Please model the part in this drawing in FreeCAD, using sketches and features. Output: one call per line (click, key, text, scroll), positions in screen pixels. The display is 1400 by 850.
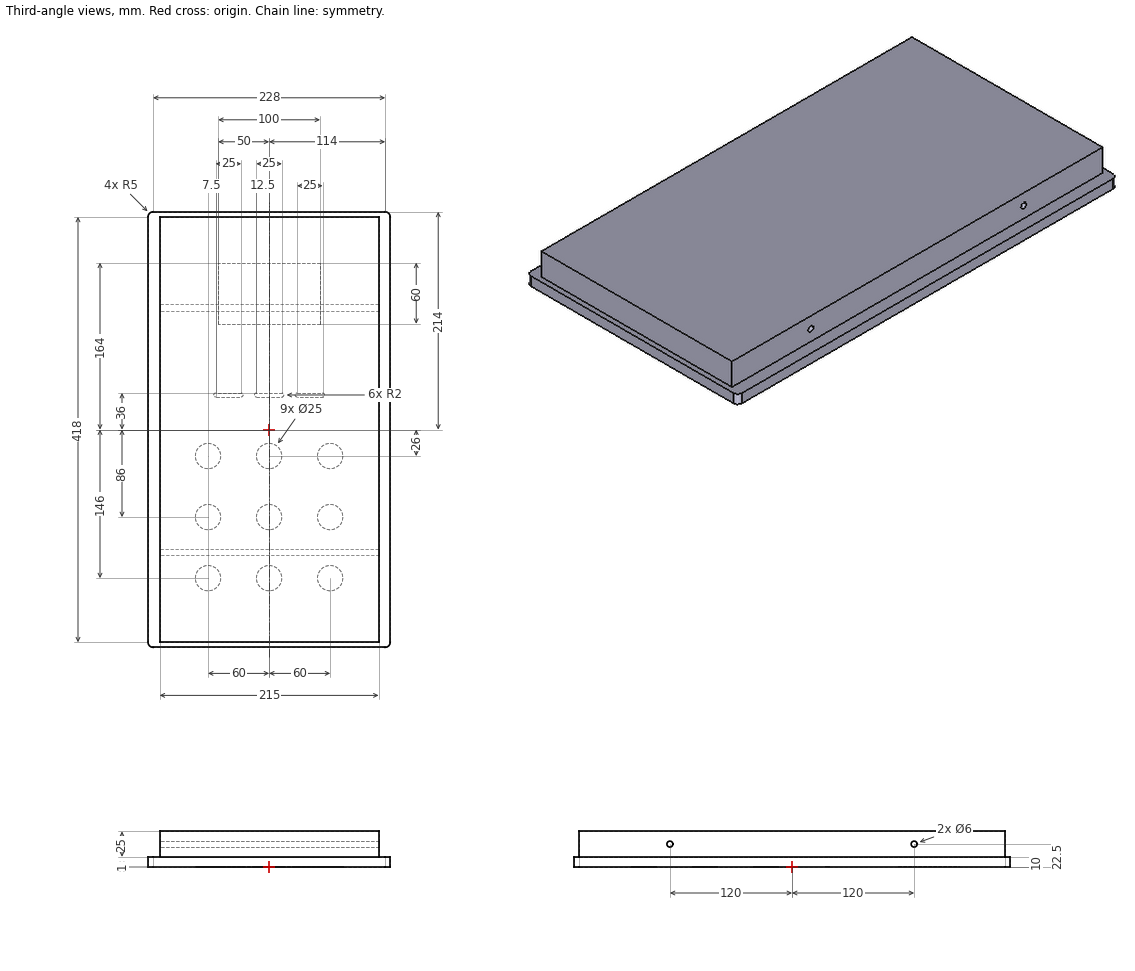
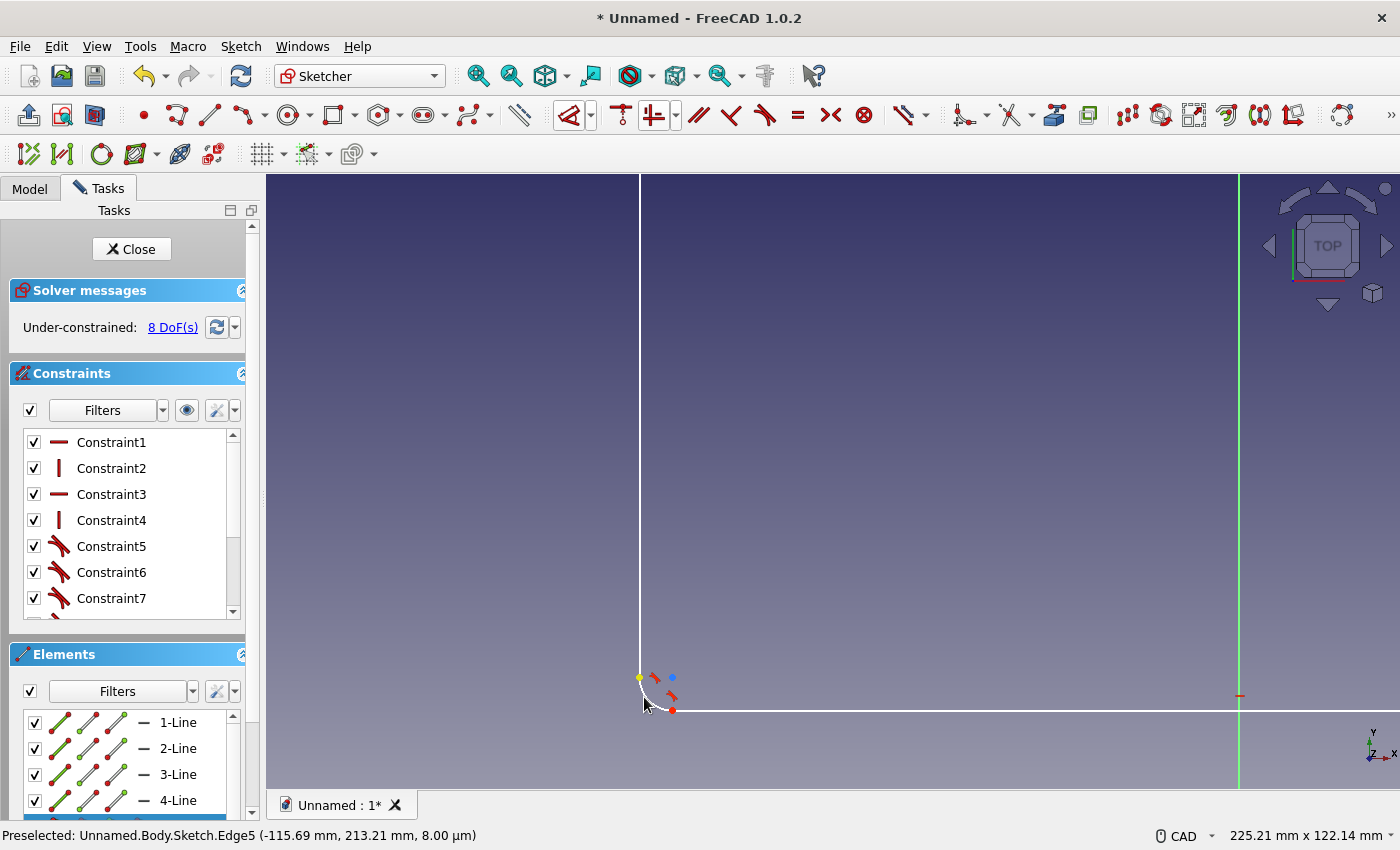
click(643, 692)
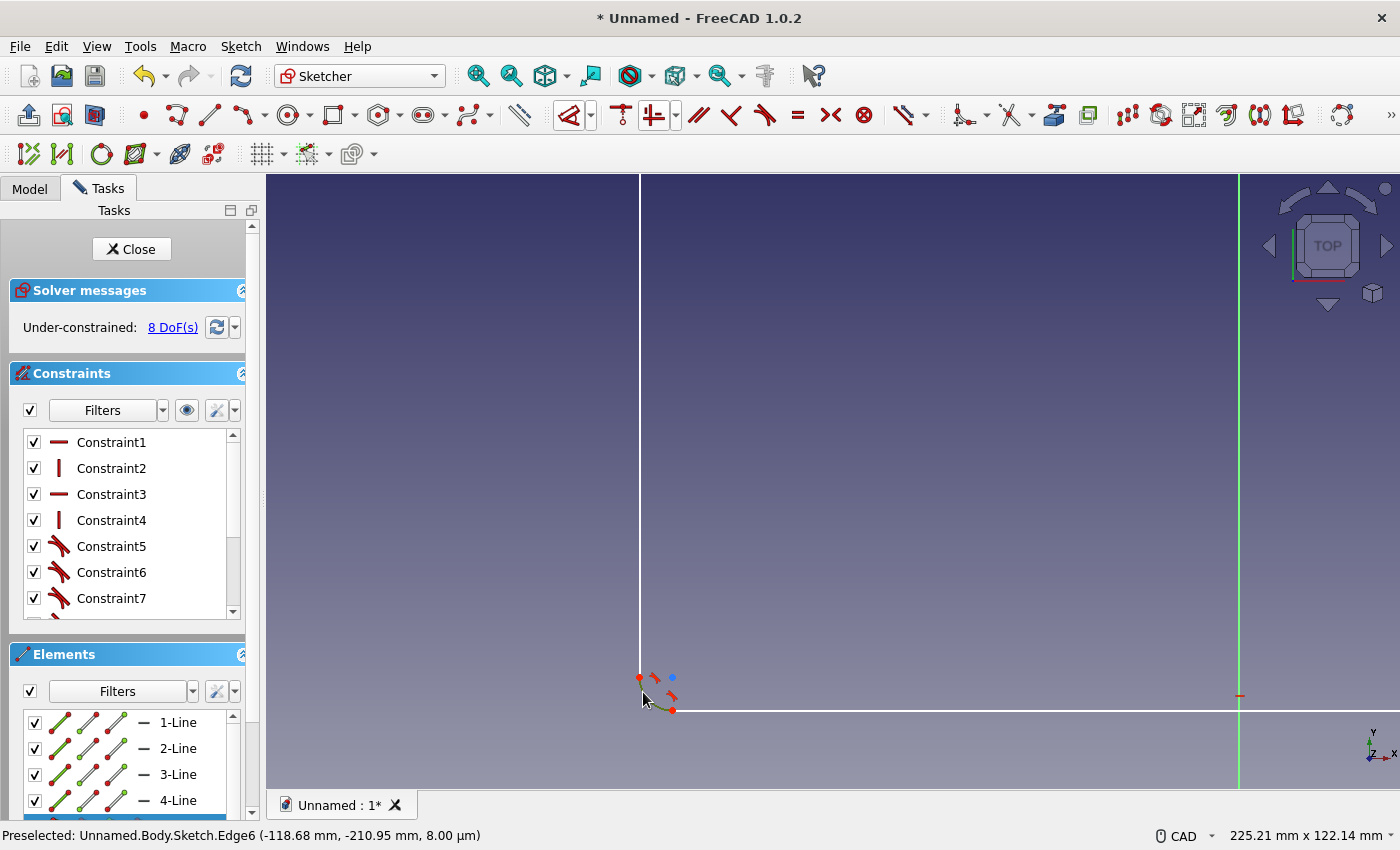
scroll(644, 698, down, 8)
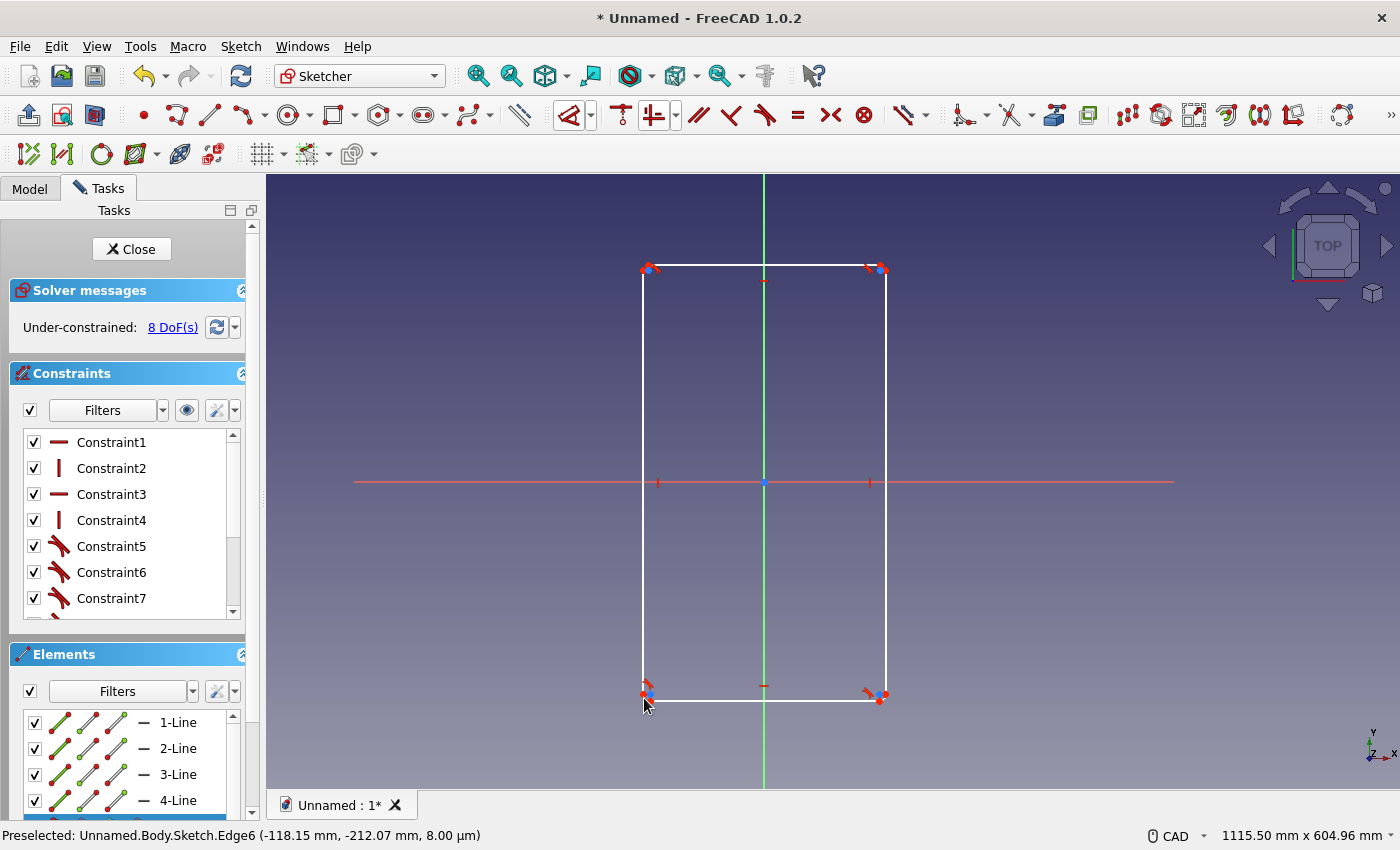
scroll(882, 701, up, 8)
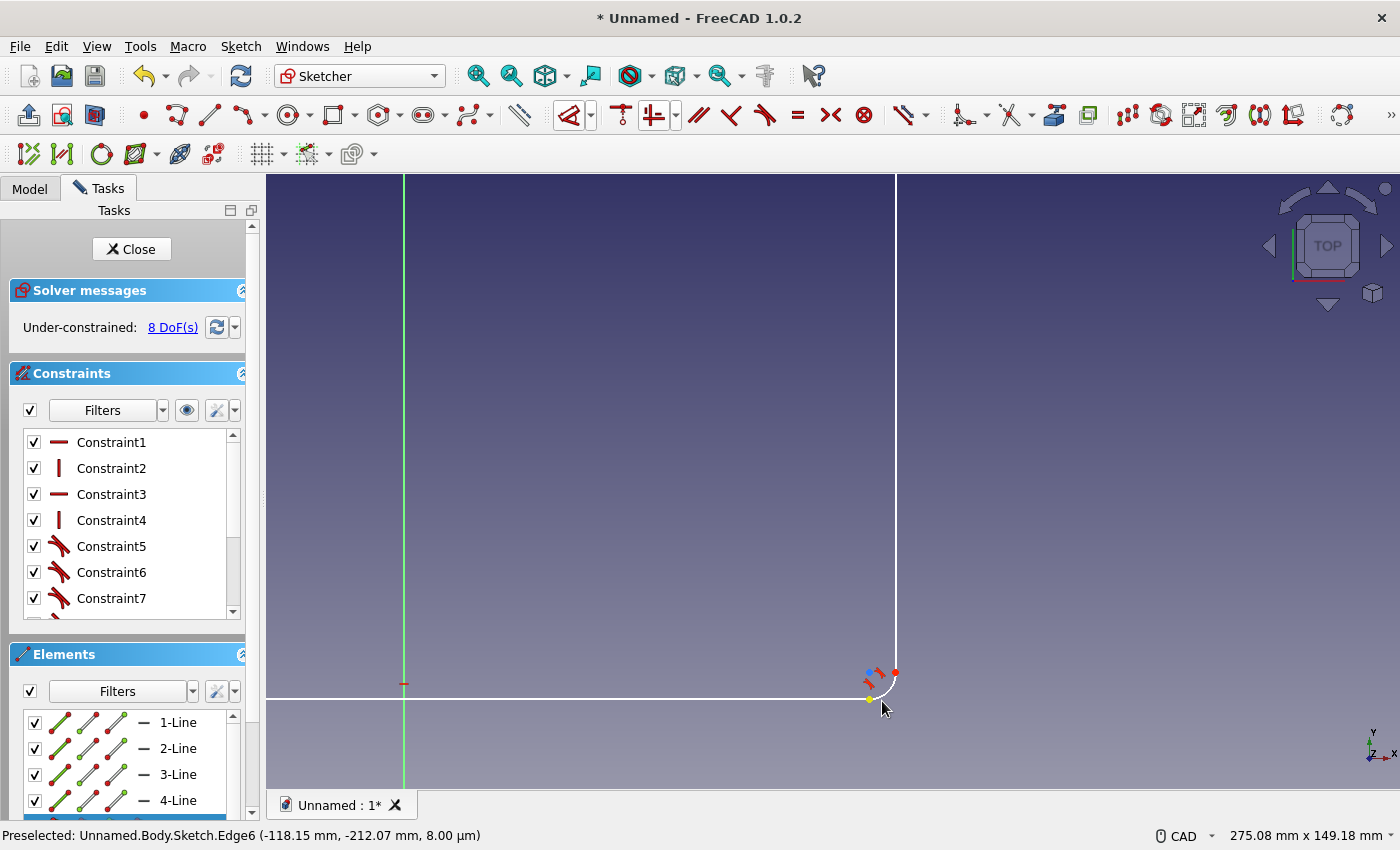
click(881, 695)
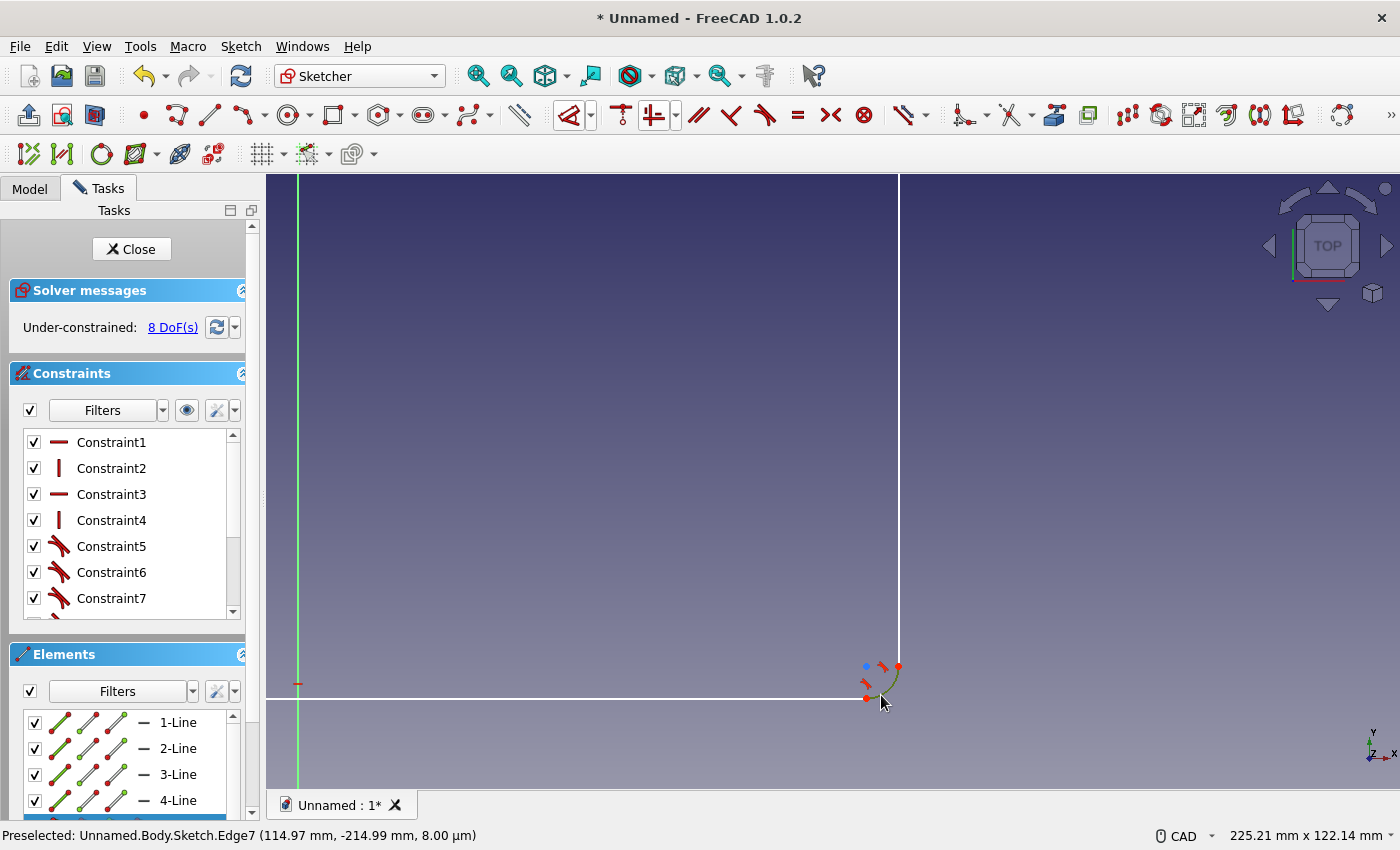
scroll(883, 701, down, 8)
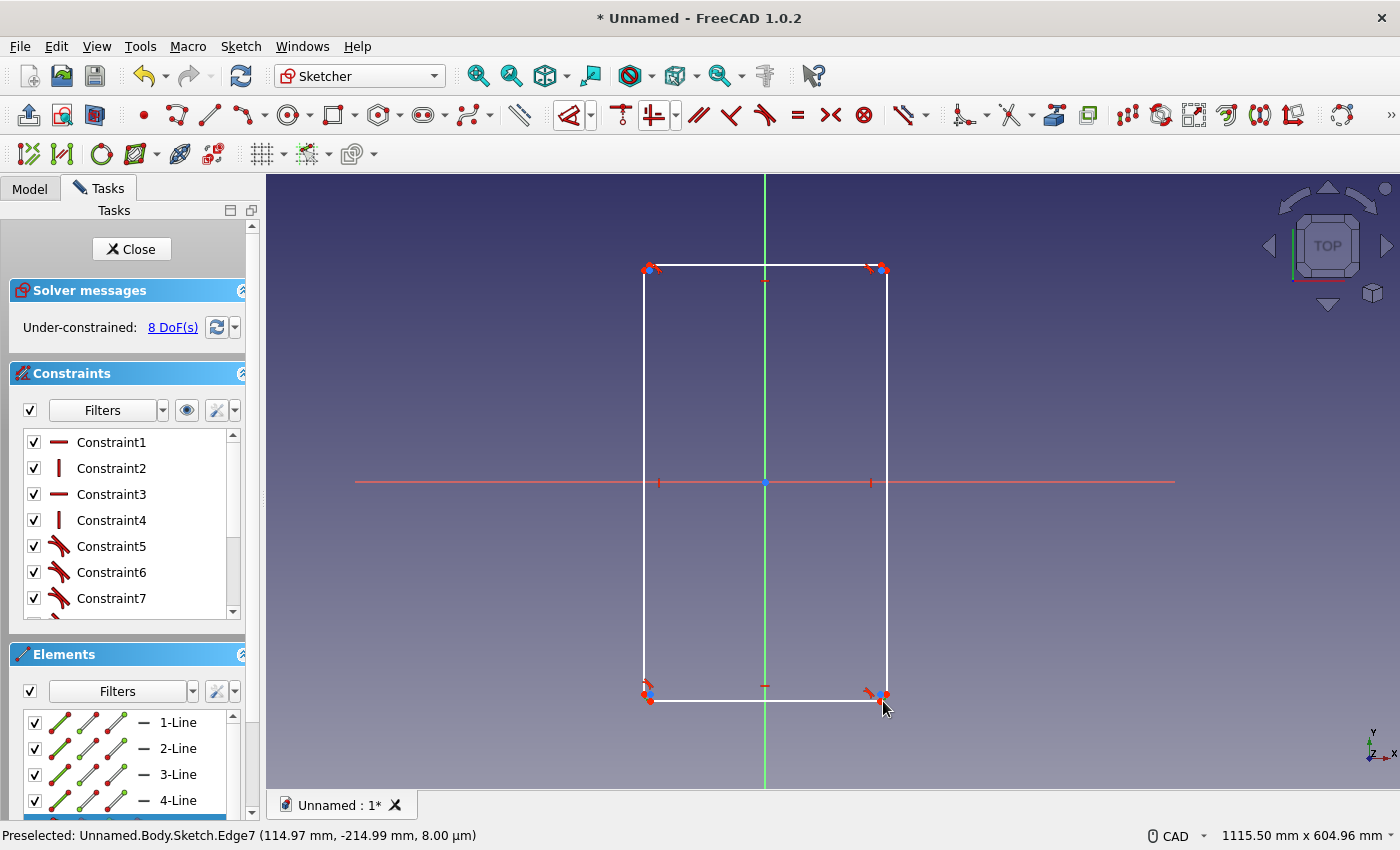
scroll(886, 268, up, 9)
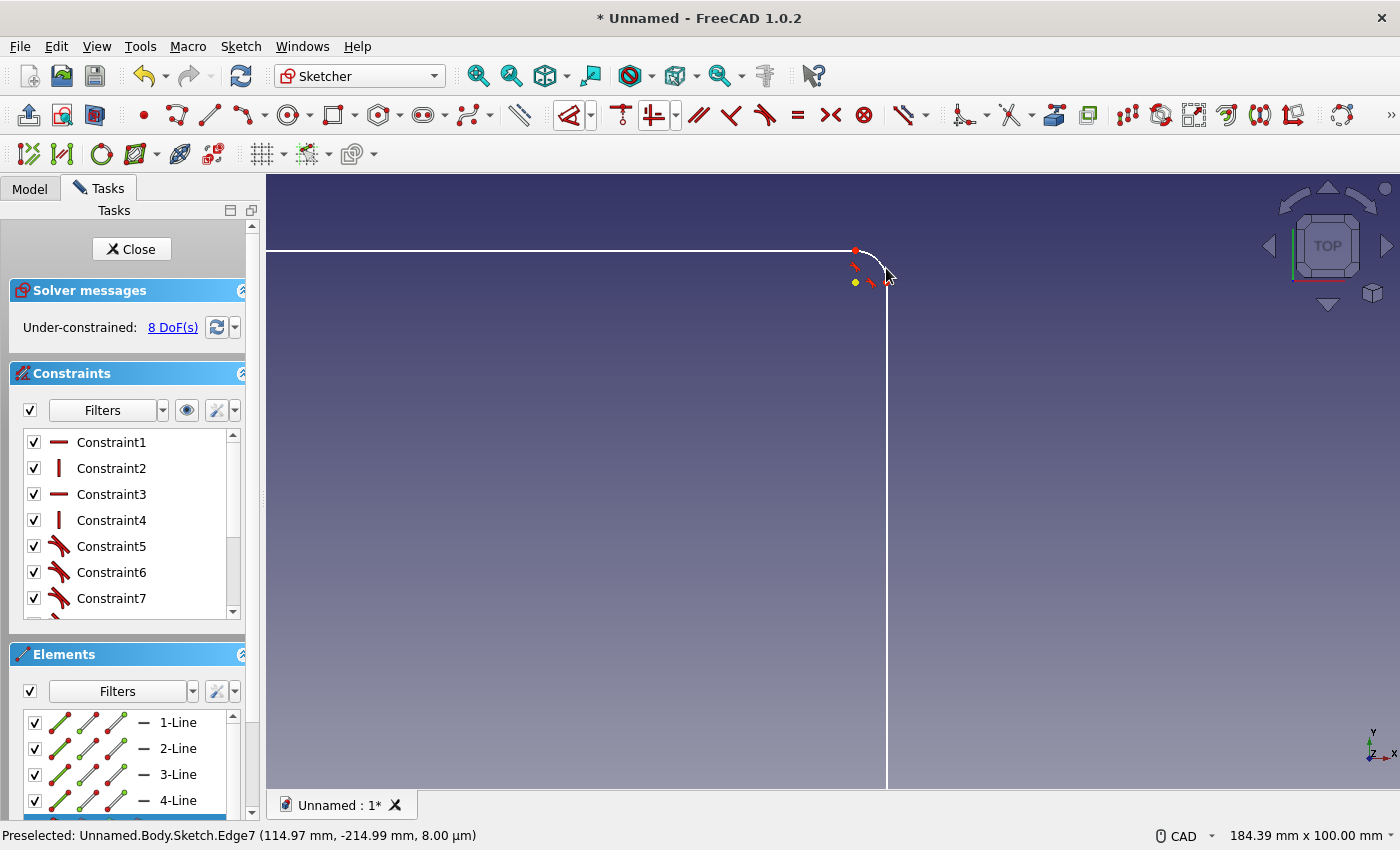
click(883, 268)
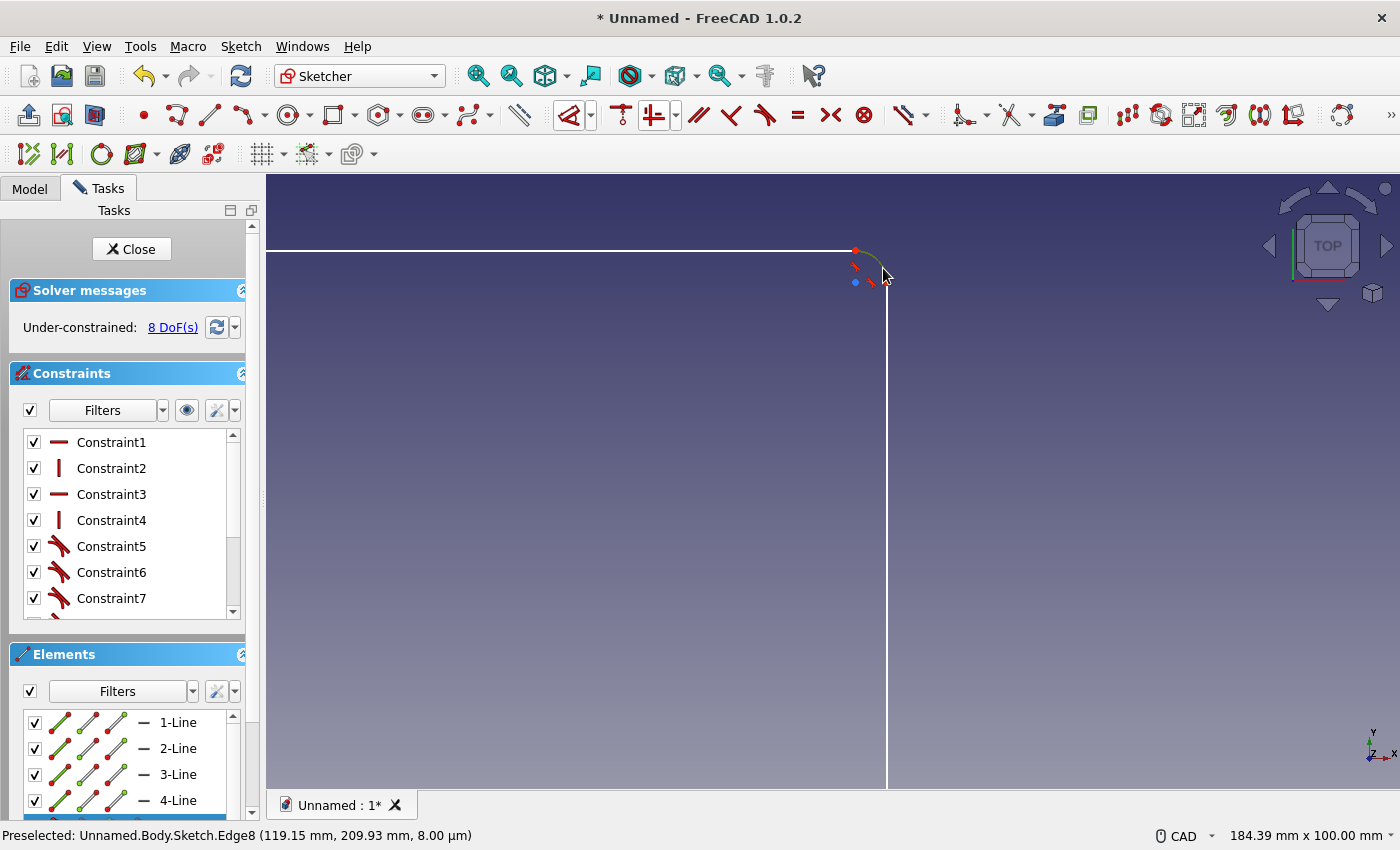
key(e)